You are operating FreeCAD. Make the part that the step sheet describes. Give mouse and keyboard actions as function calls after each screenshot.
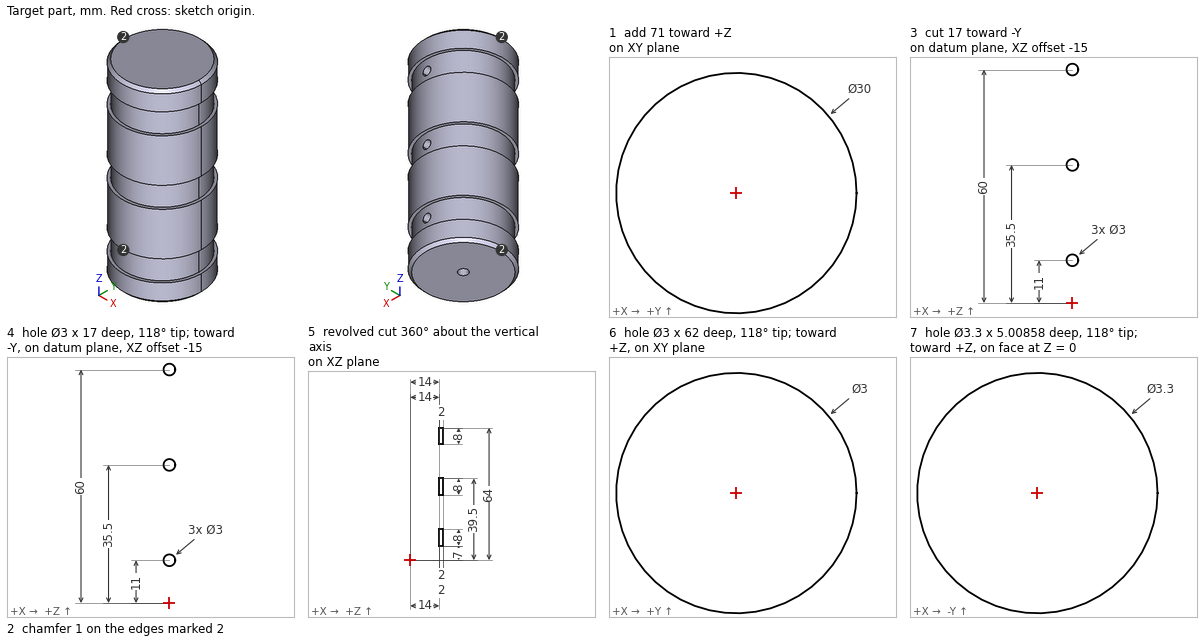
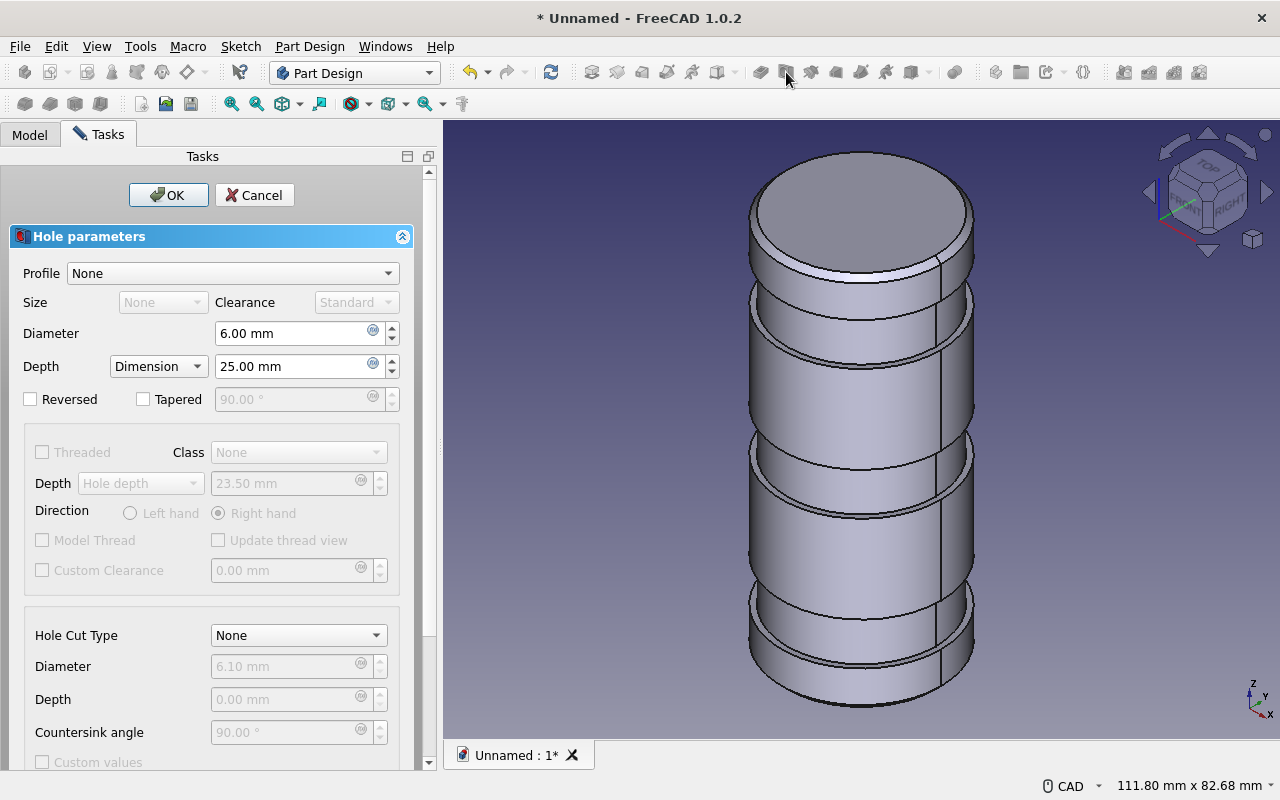
triple_click(300, 334)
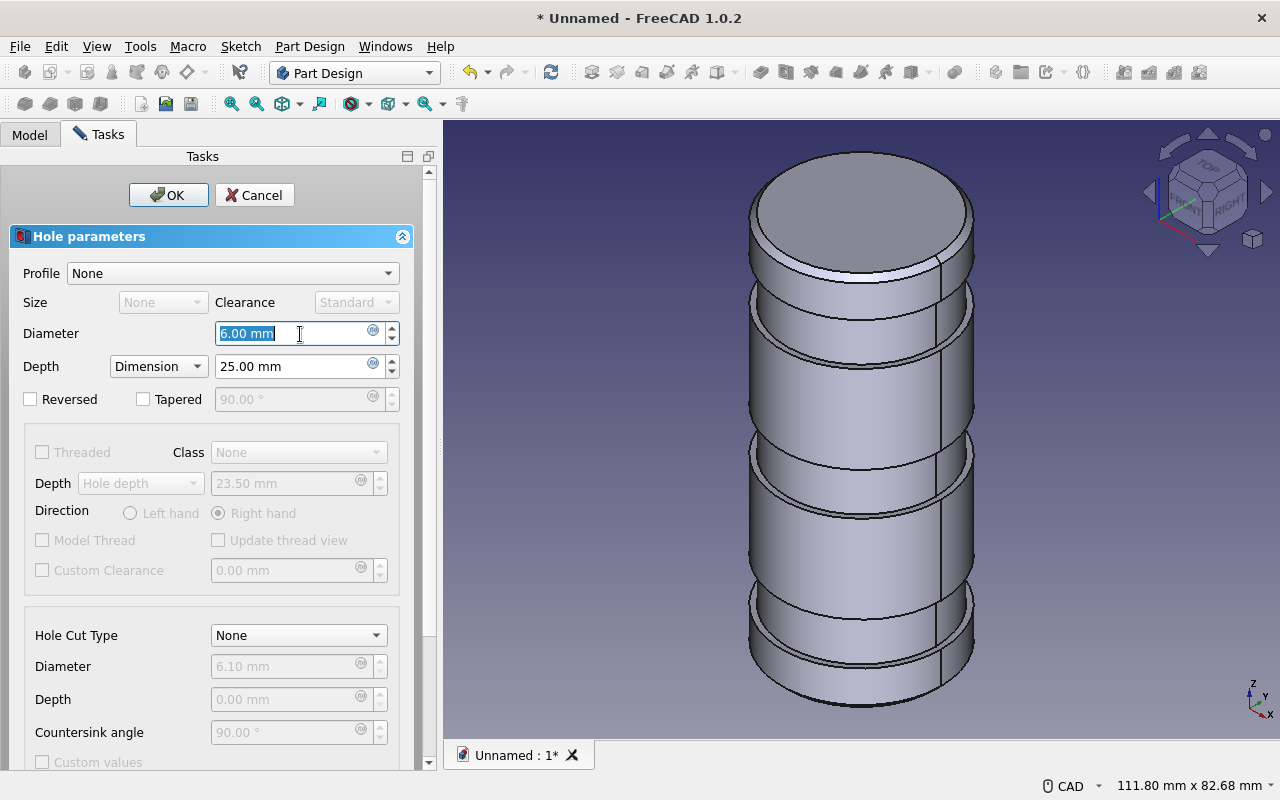
text(3)
key(Tab)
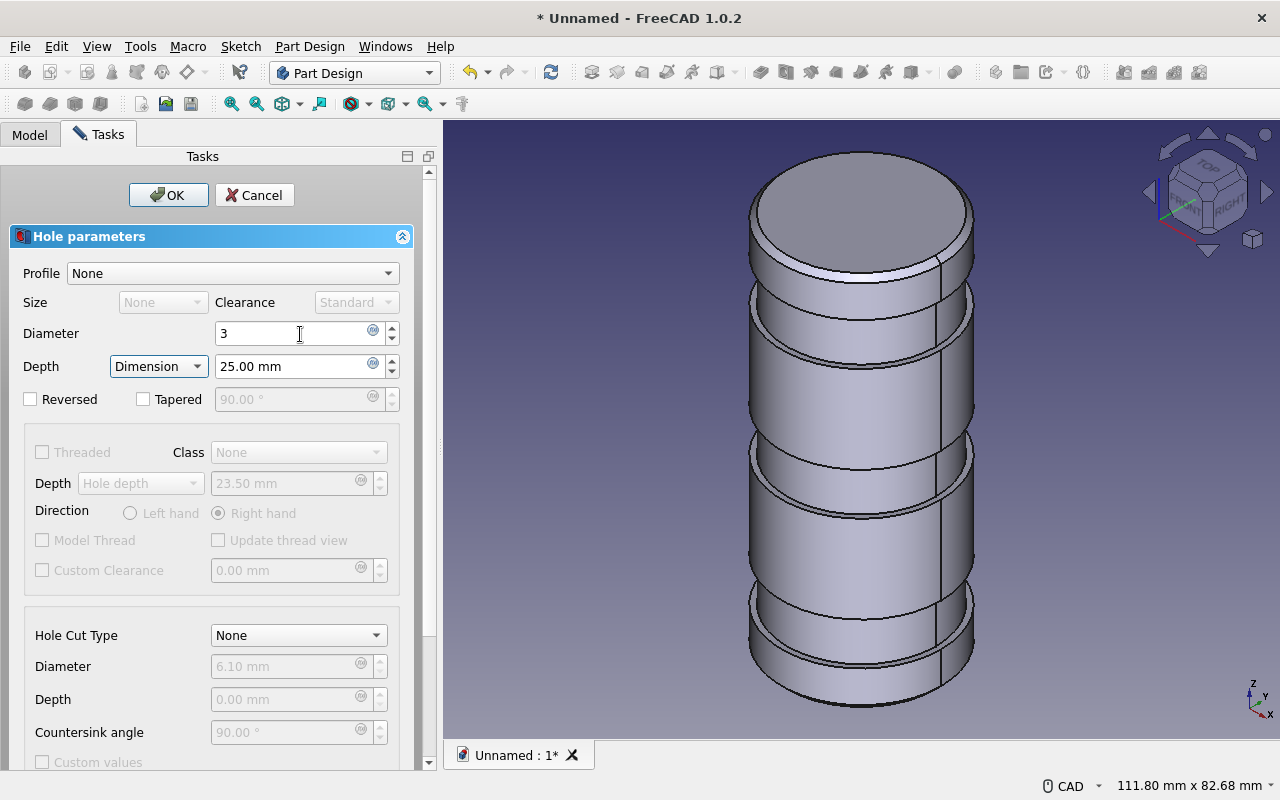
triple_click(300, 366)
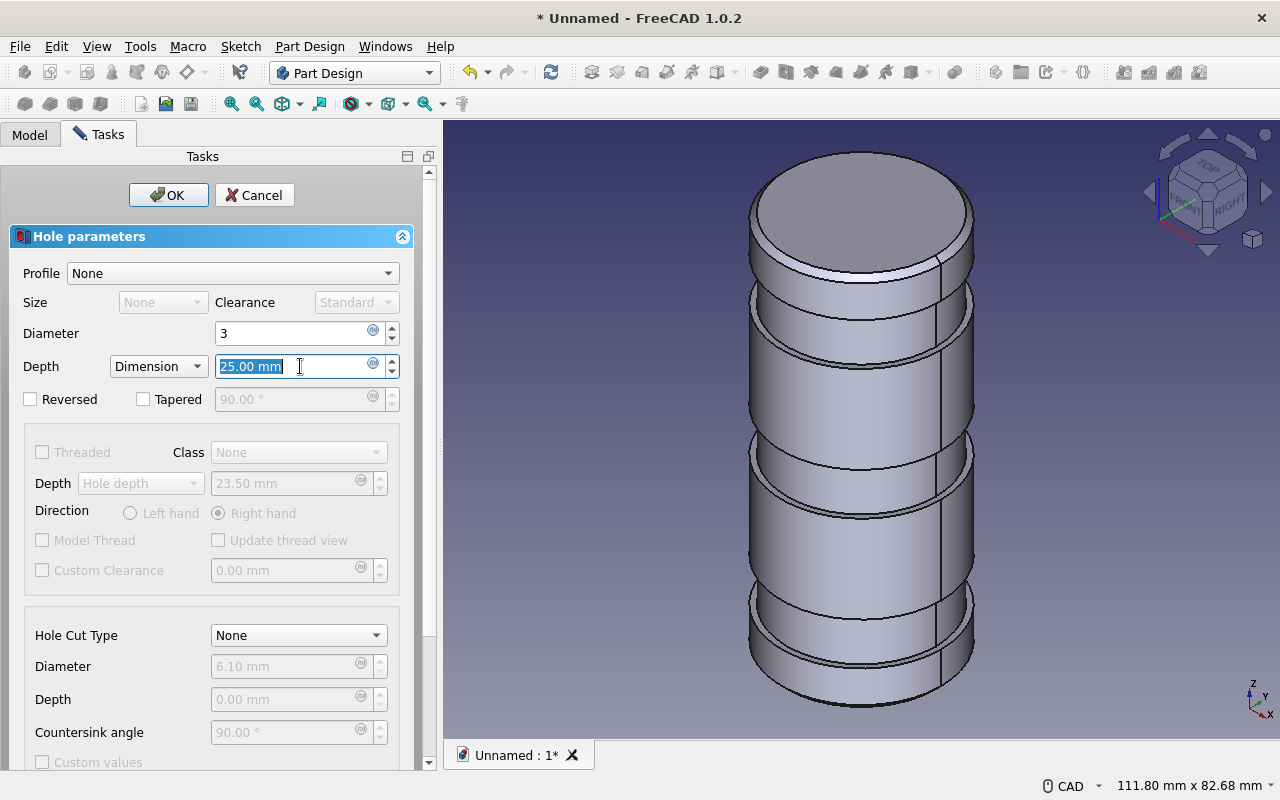
text(62)
key(Tab)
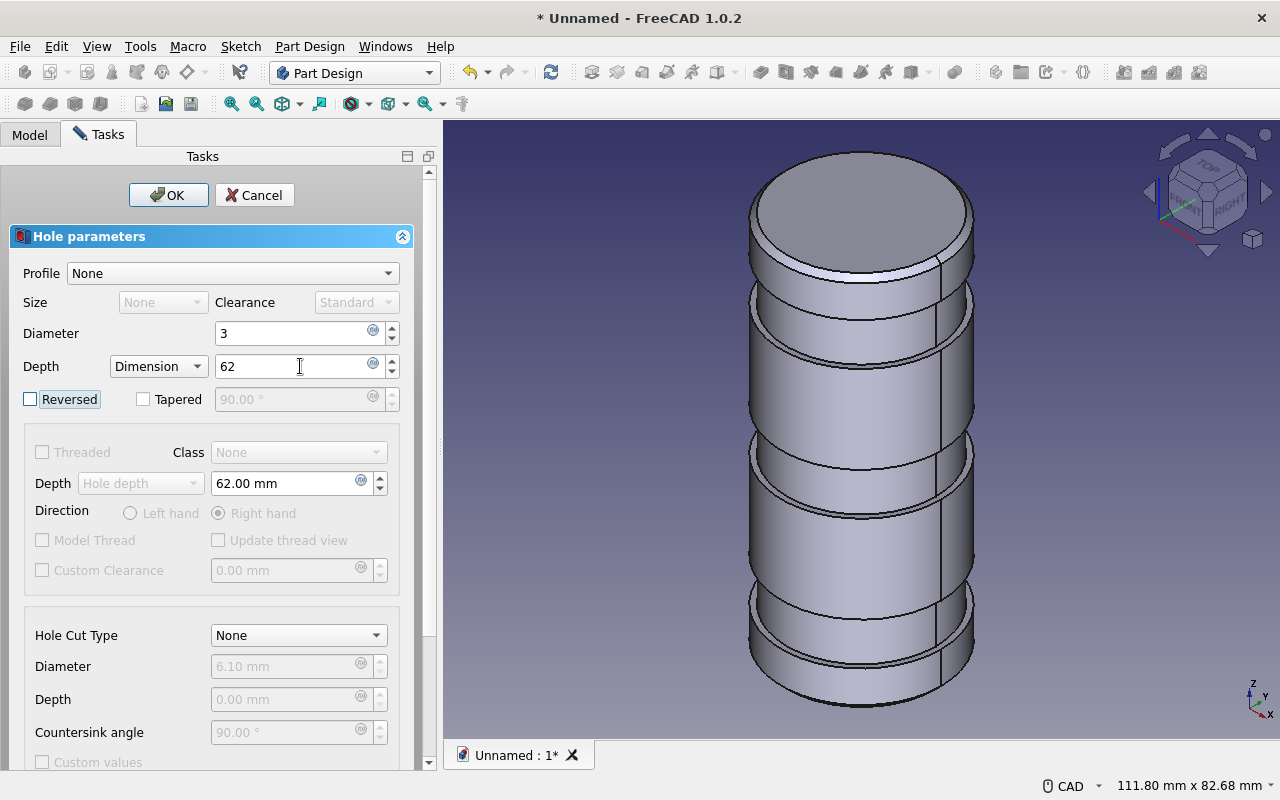
click(31, 399)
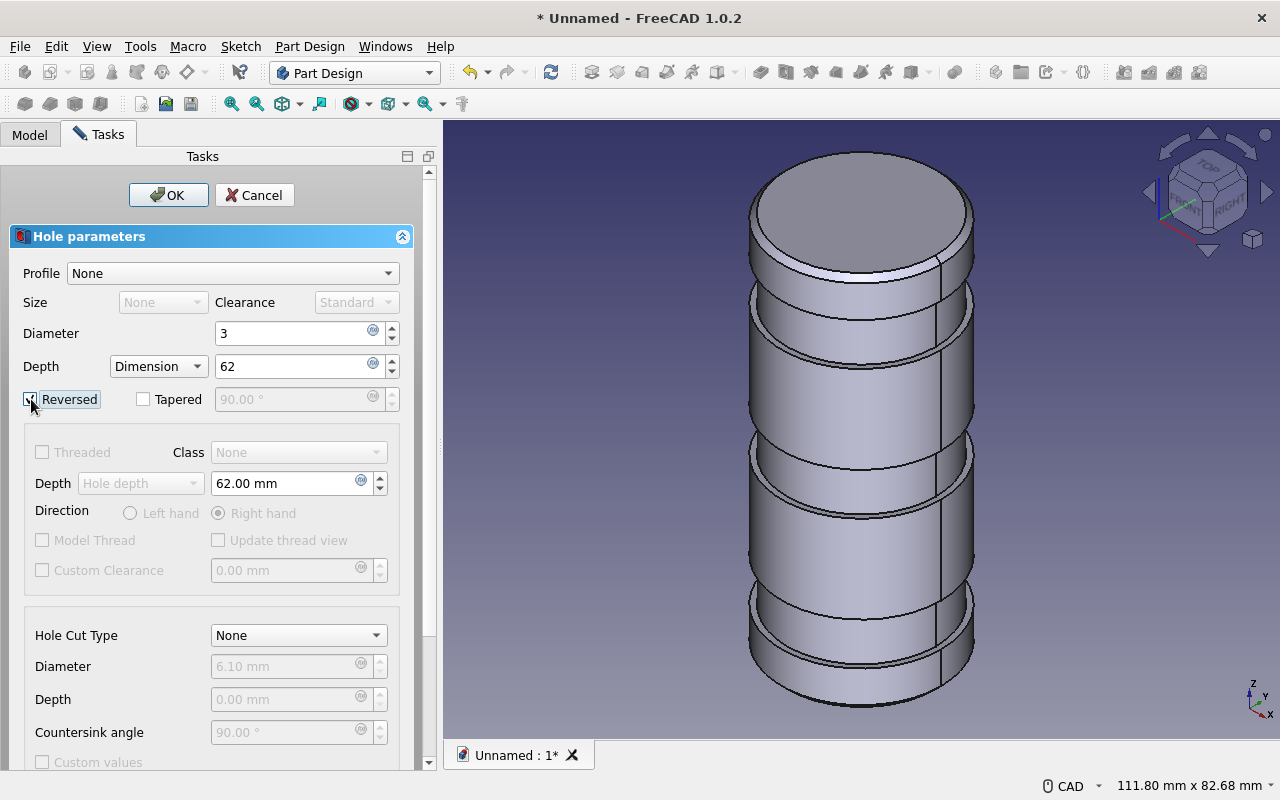
click(169, 195)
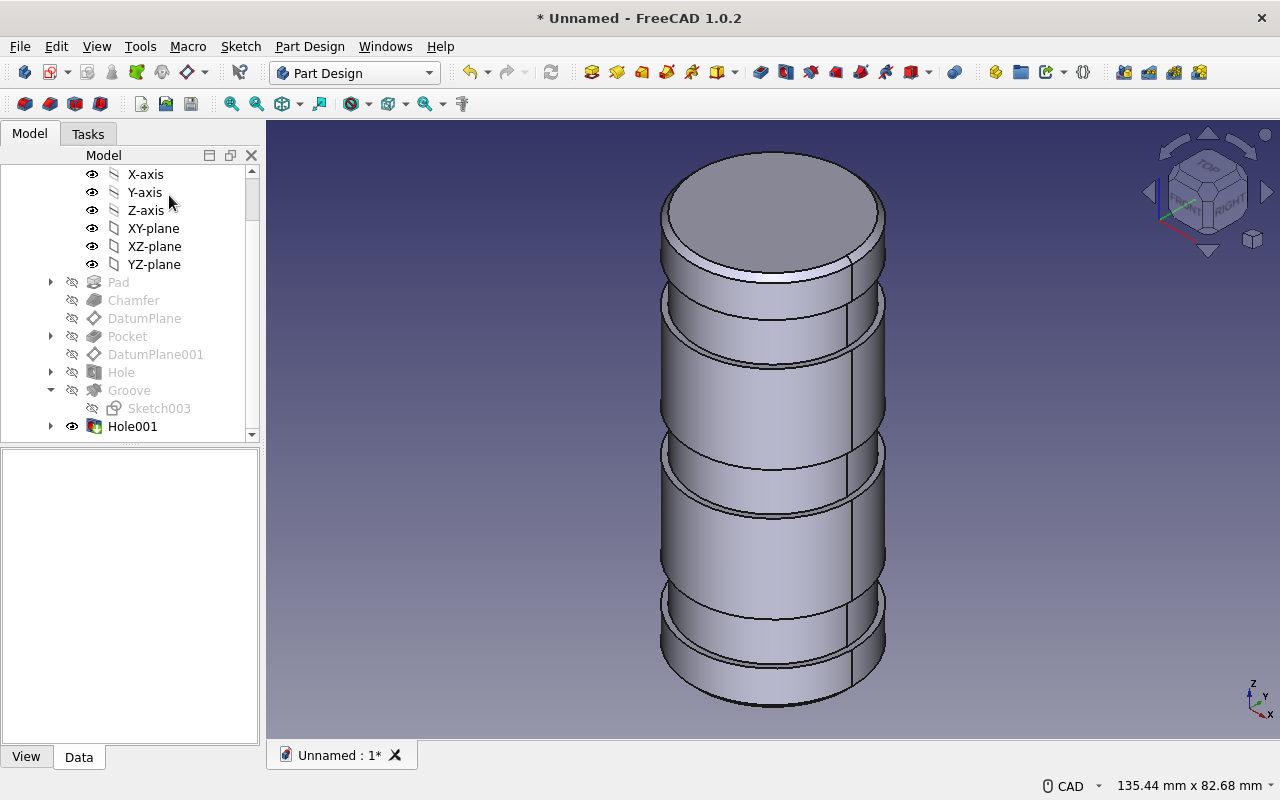
key(5)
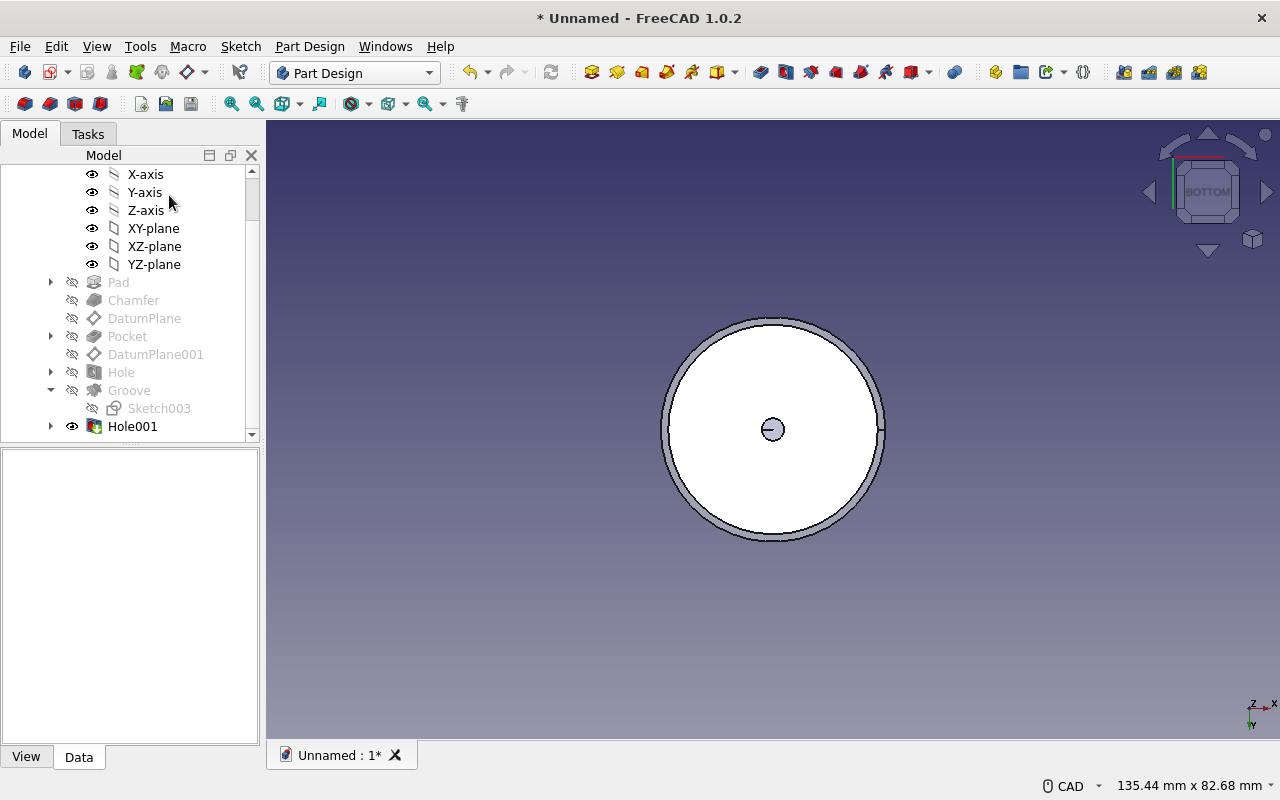
click(232, 104)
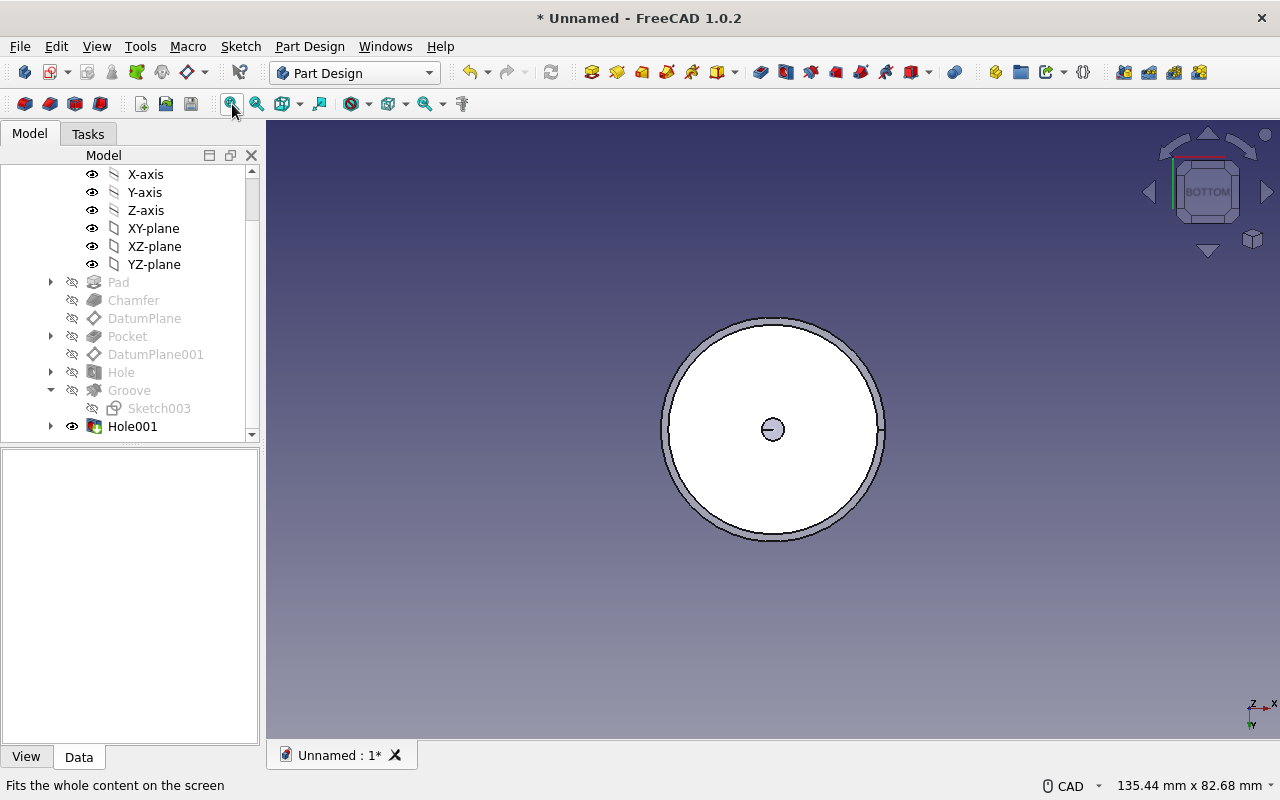
click(833, 428)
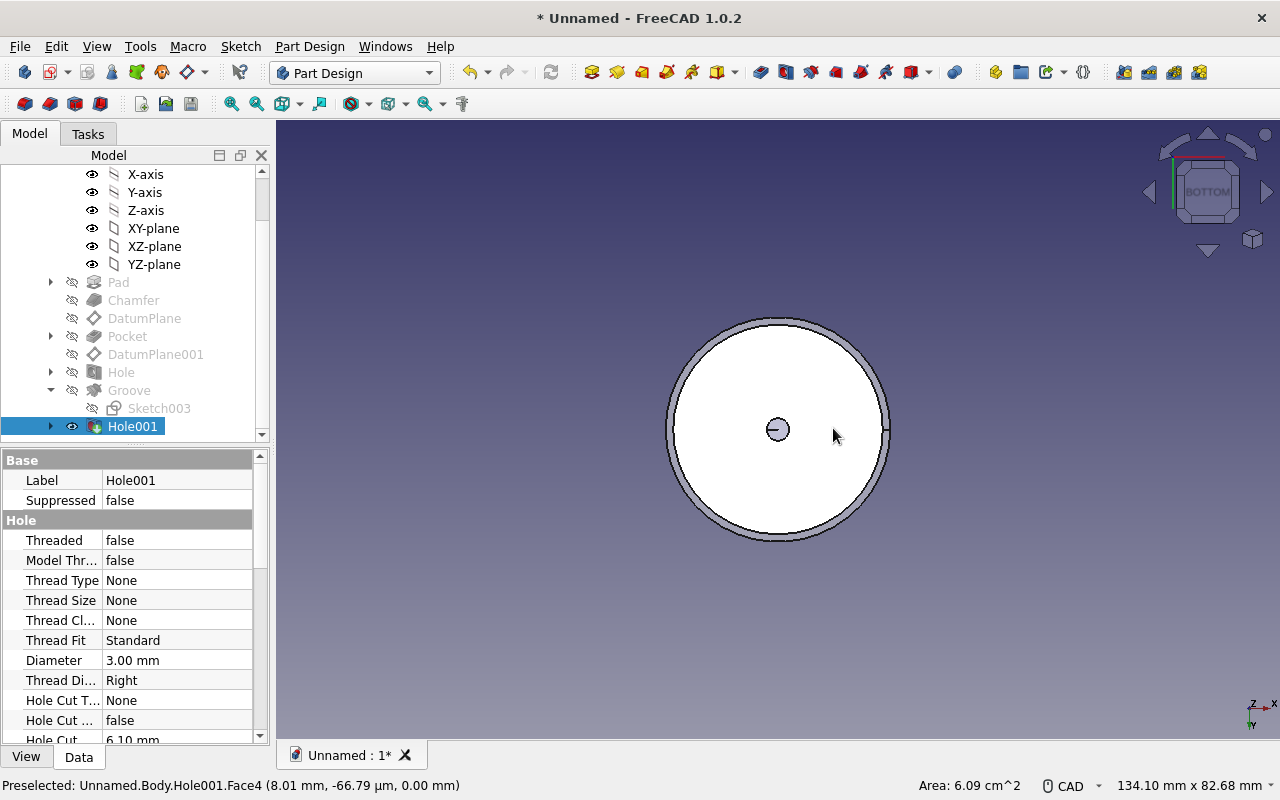
click(50, 72)